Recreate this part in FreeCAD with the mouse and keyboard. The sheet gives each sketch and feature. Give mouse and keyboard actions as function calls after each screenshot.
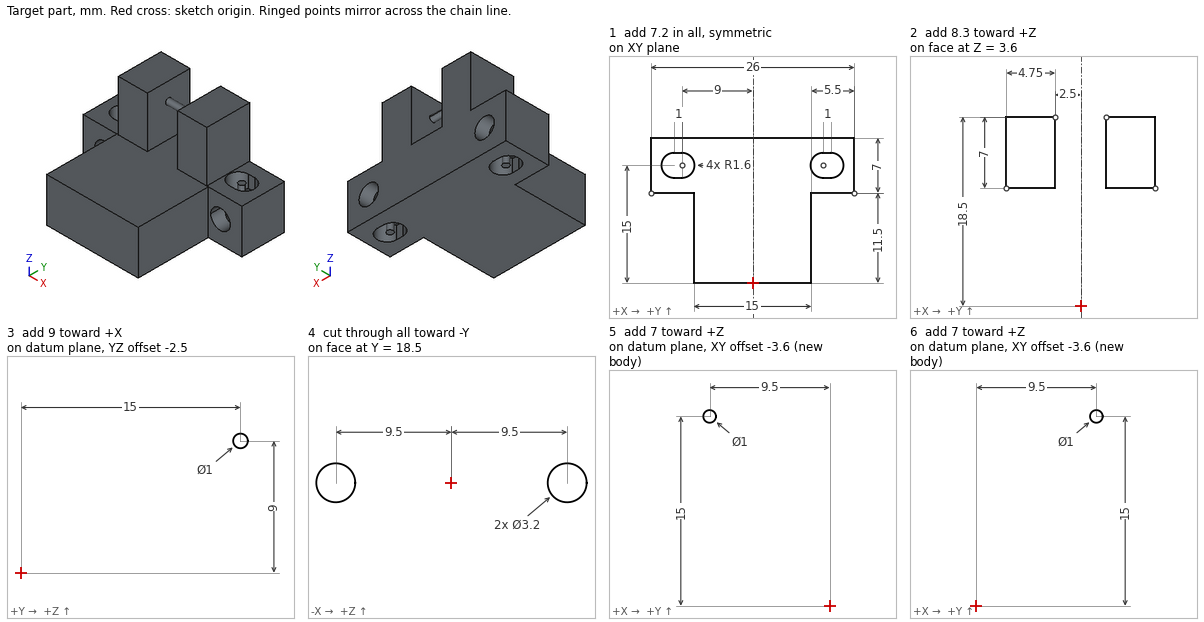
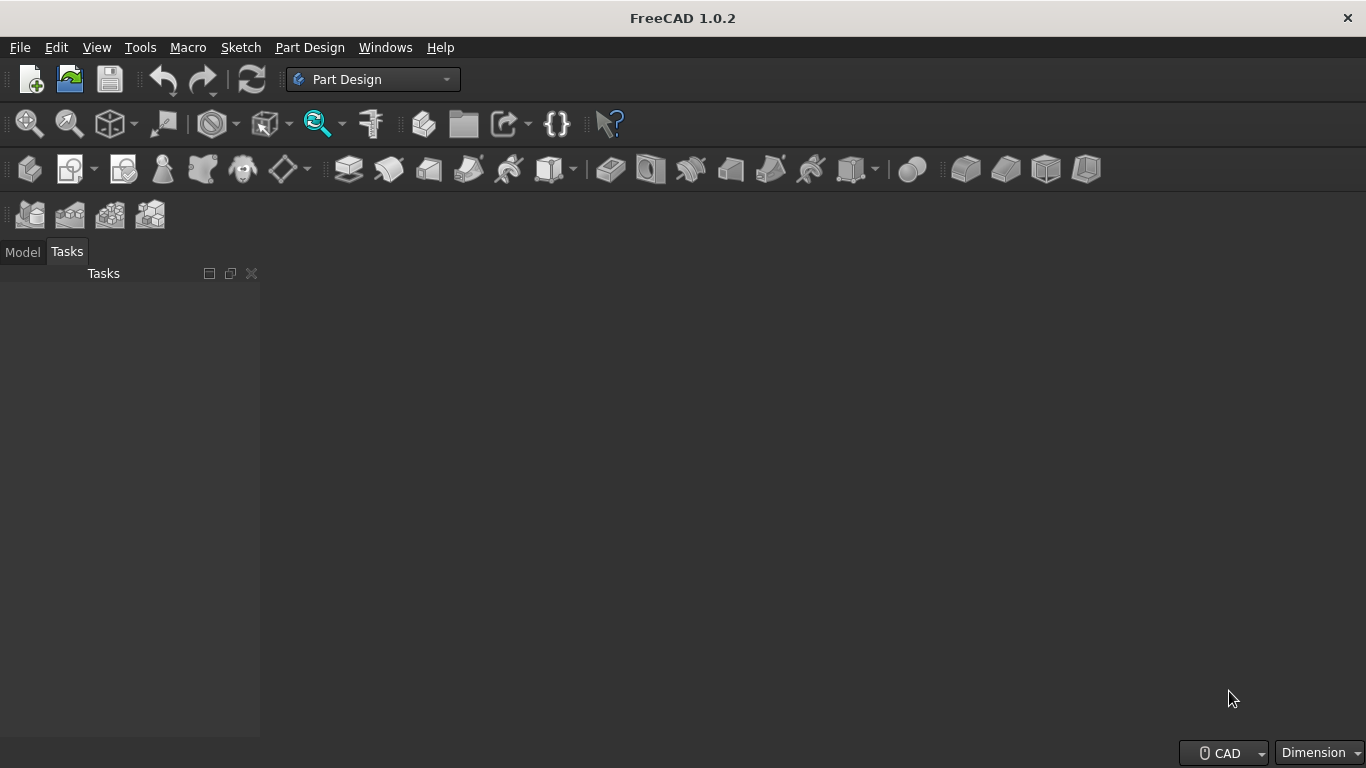
click(30, 80)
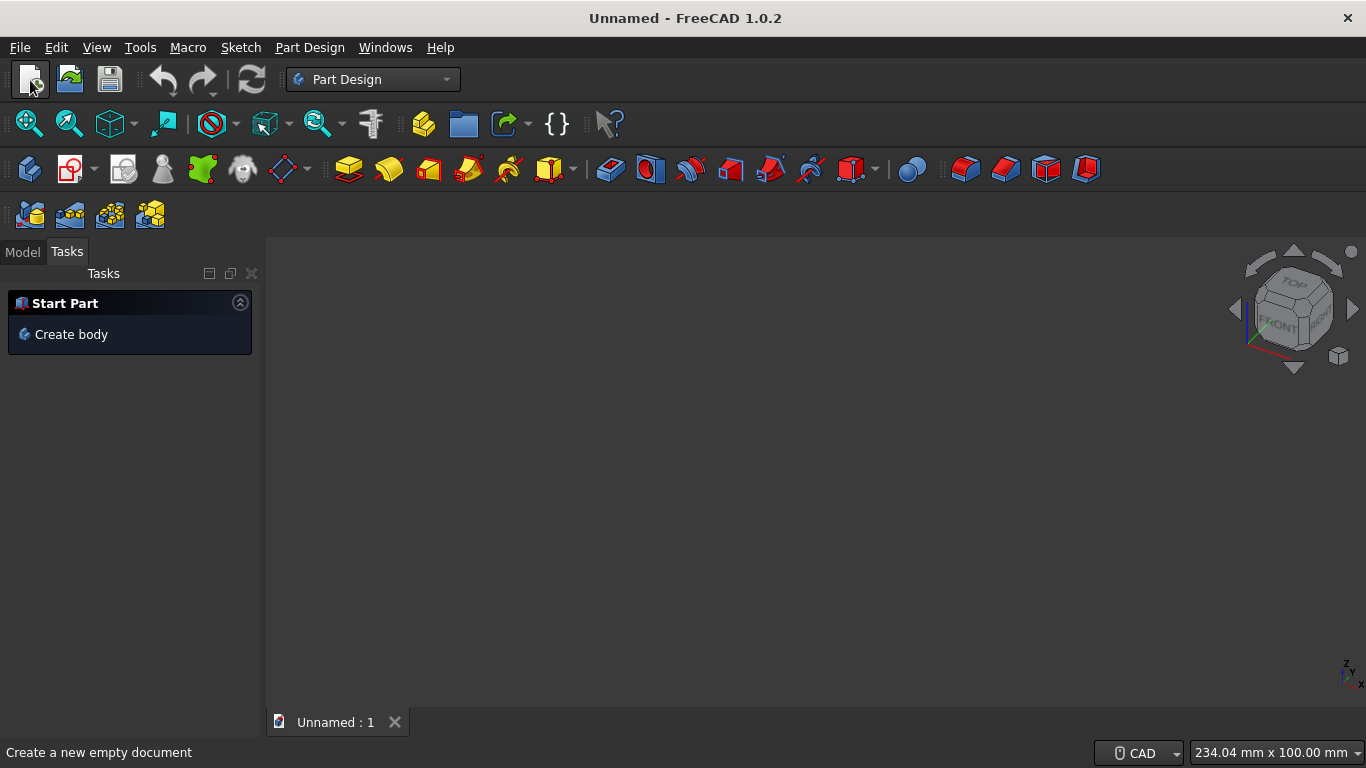
click(70, 170)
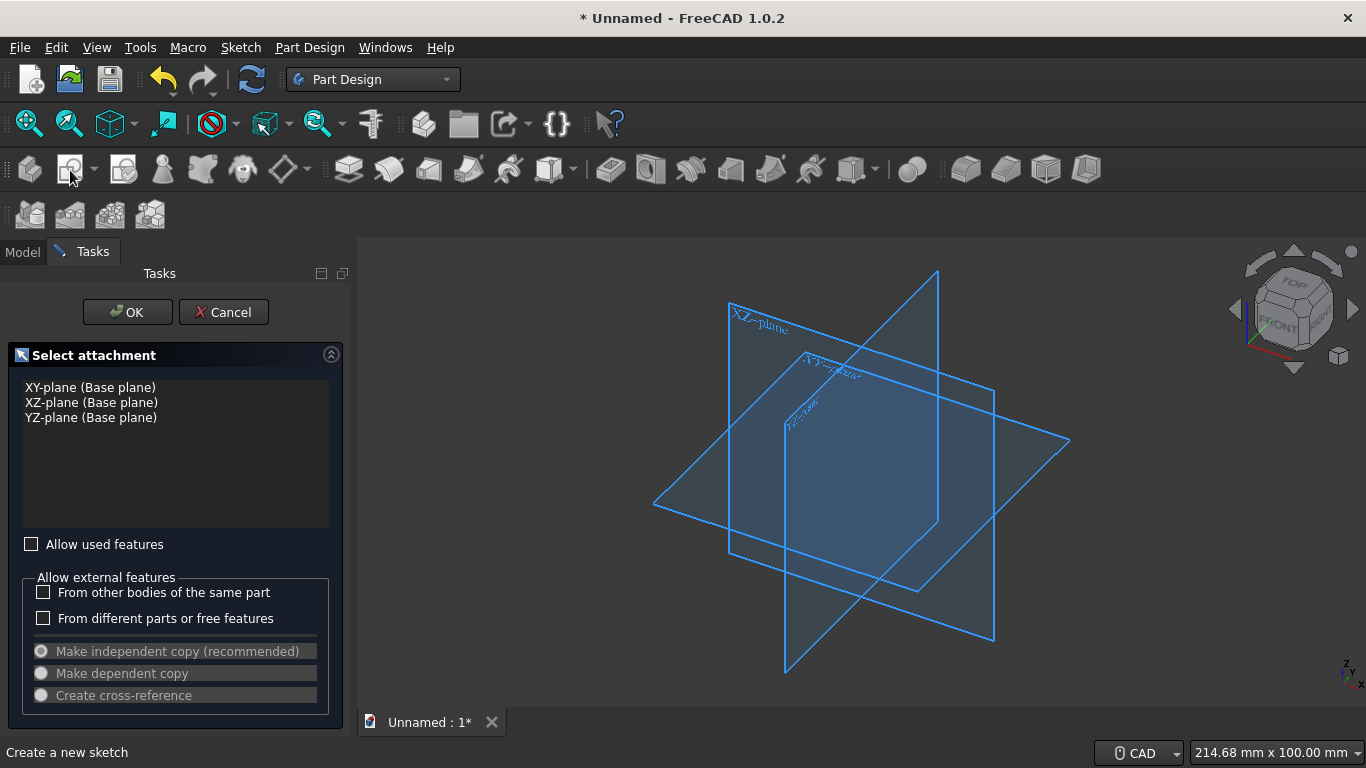
click(82, 388)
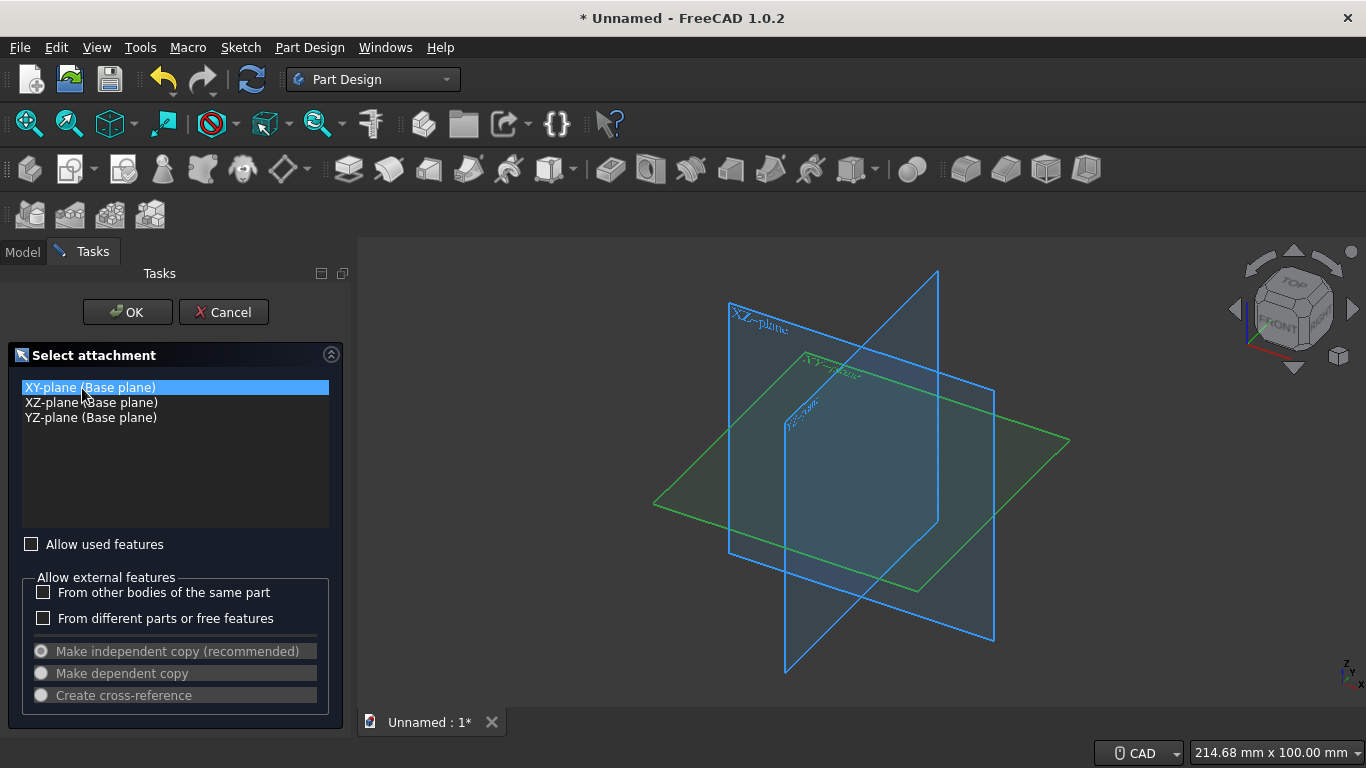
click(128, 312)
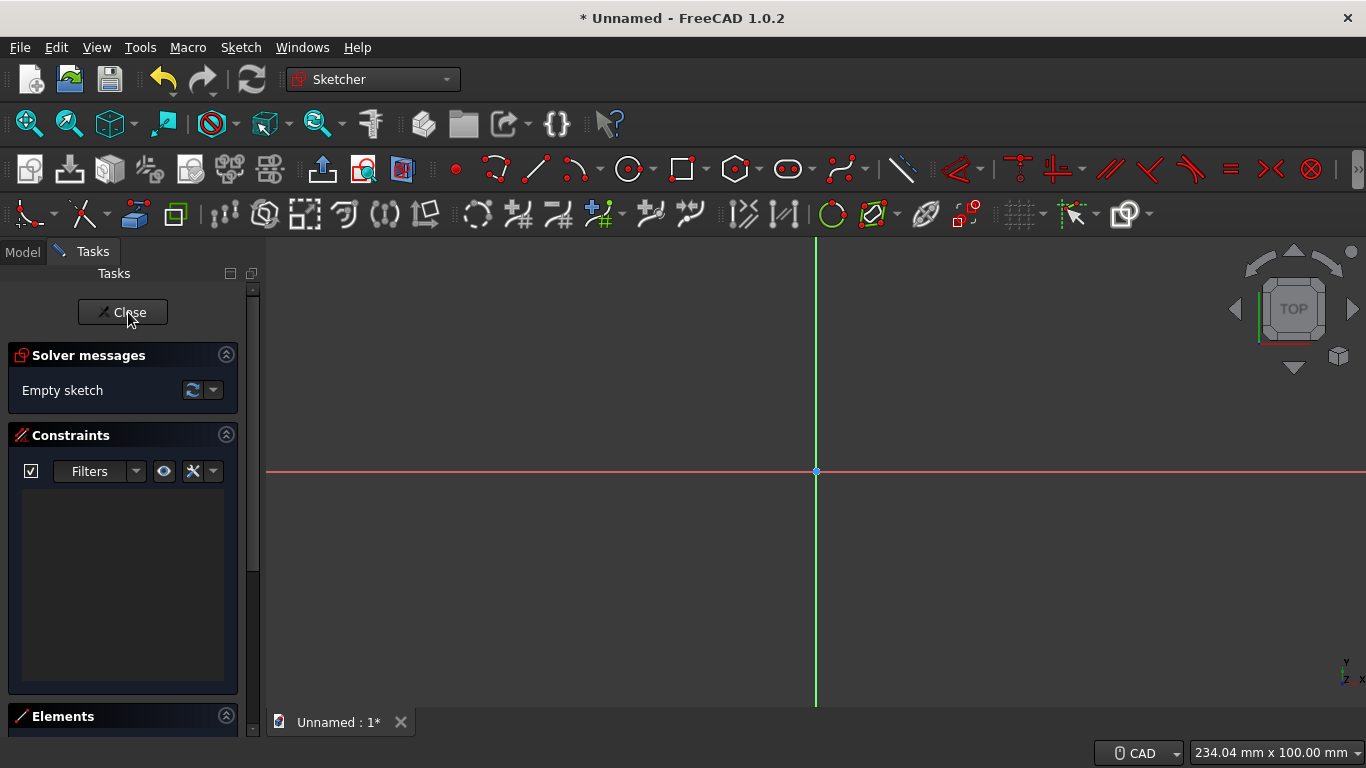
scroll(846, 410, up, 6)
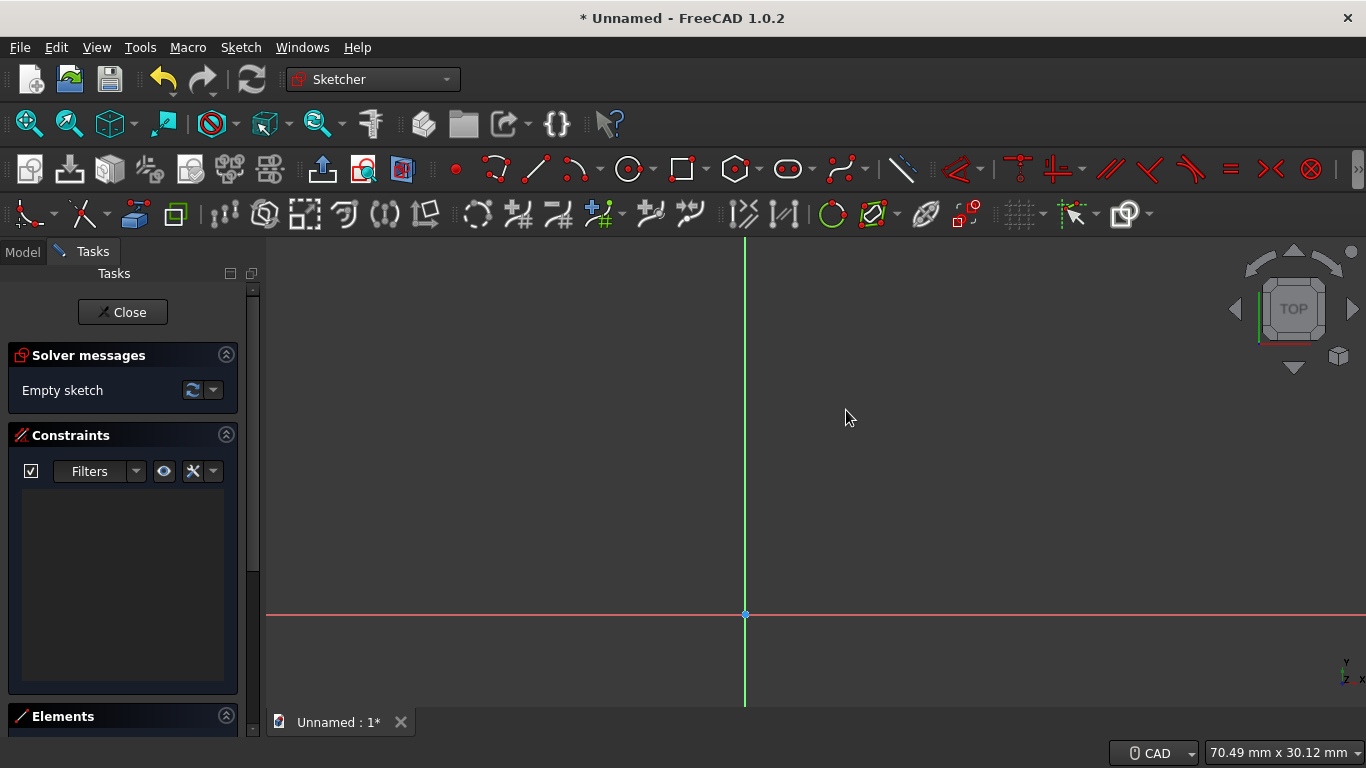
key(g)
key(m)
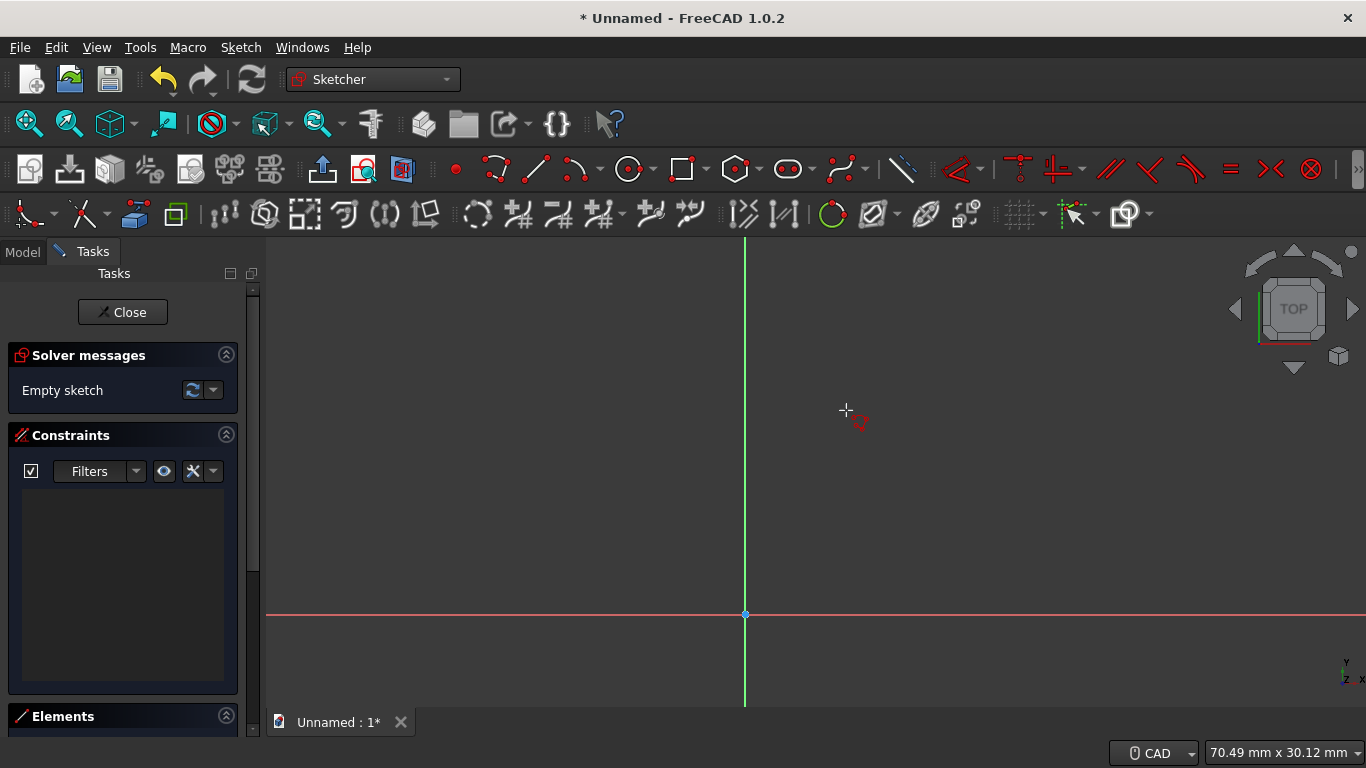
click(628, 615)
click(862, 606)
click(862, 436)
click(948, 436)
click(948, 326)
click(542, 326)
click(542, 436)
click(628, 436)
click(628, 615)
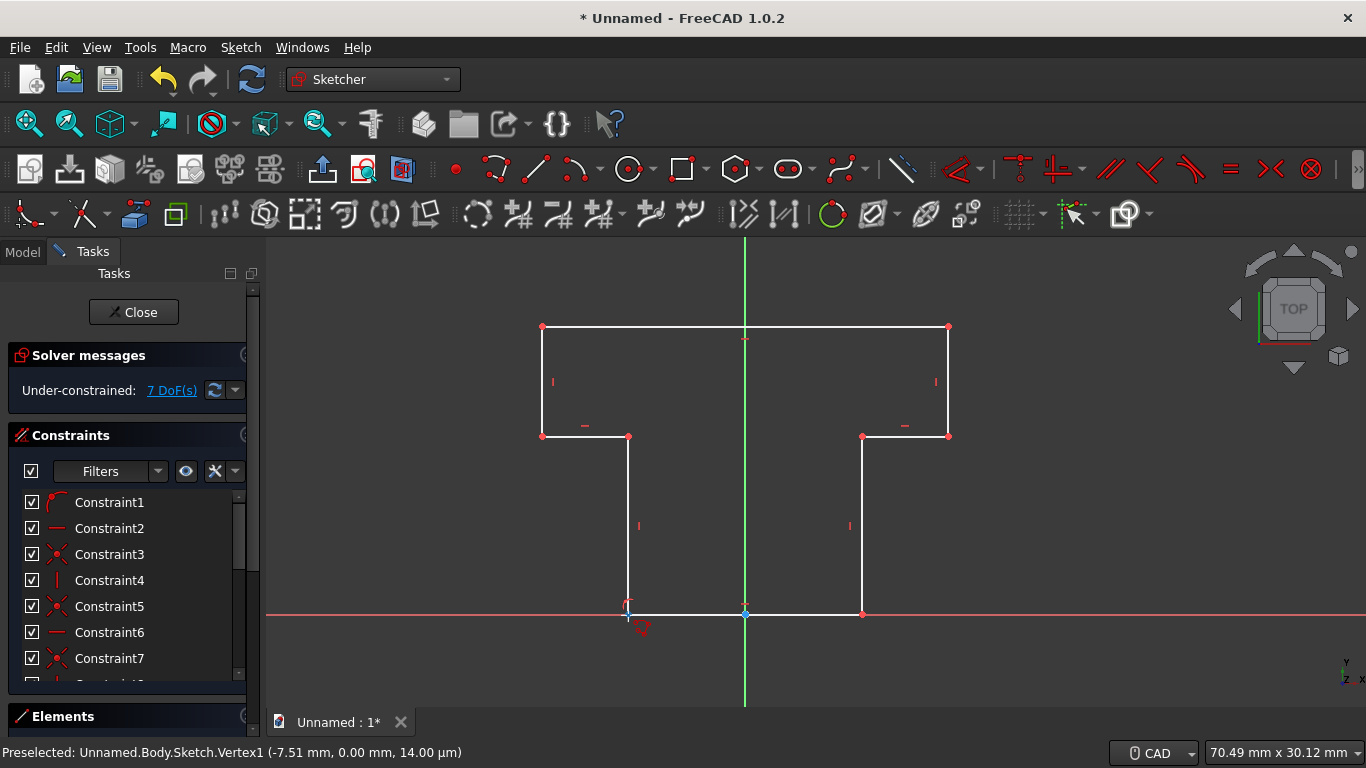
key(g)
key(s)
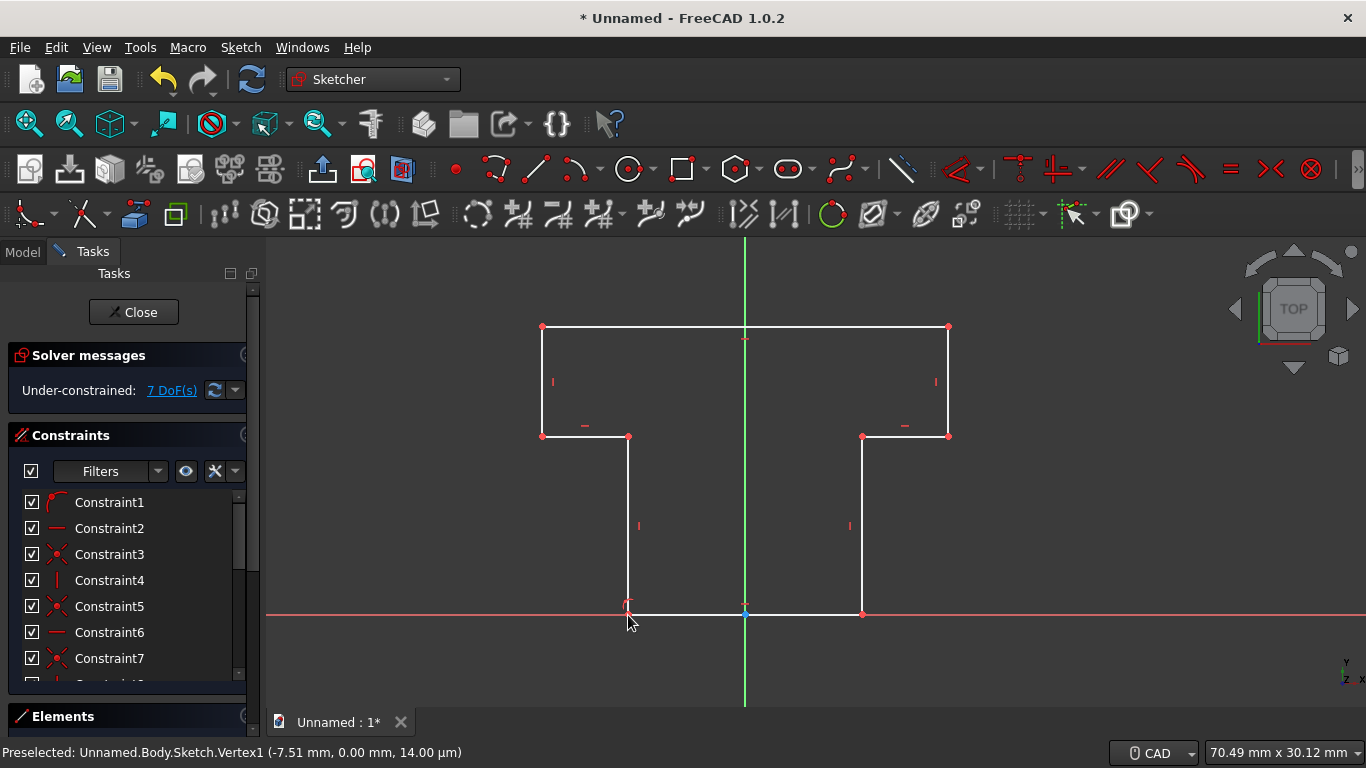
click(589, 381)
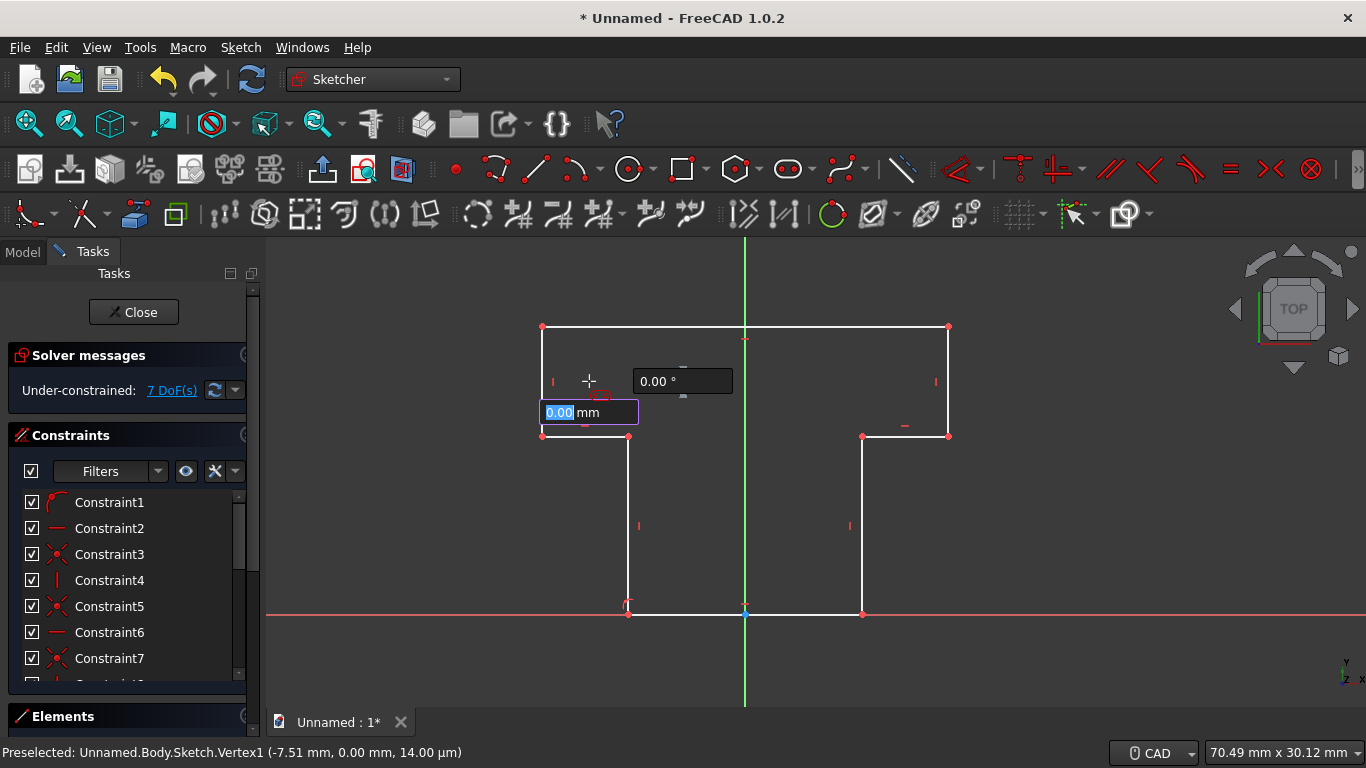
click(605, 381)